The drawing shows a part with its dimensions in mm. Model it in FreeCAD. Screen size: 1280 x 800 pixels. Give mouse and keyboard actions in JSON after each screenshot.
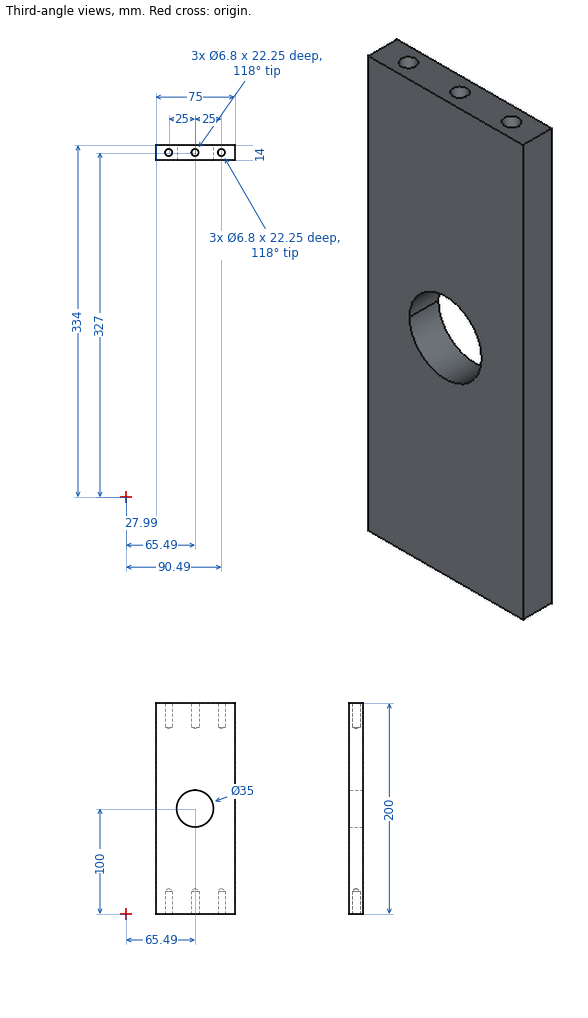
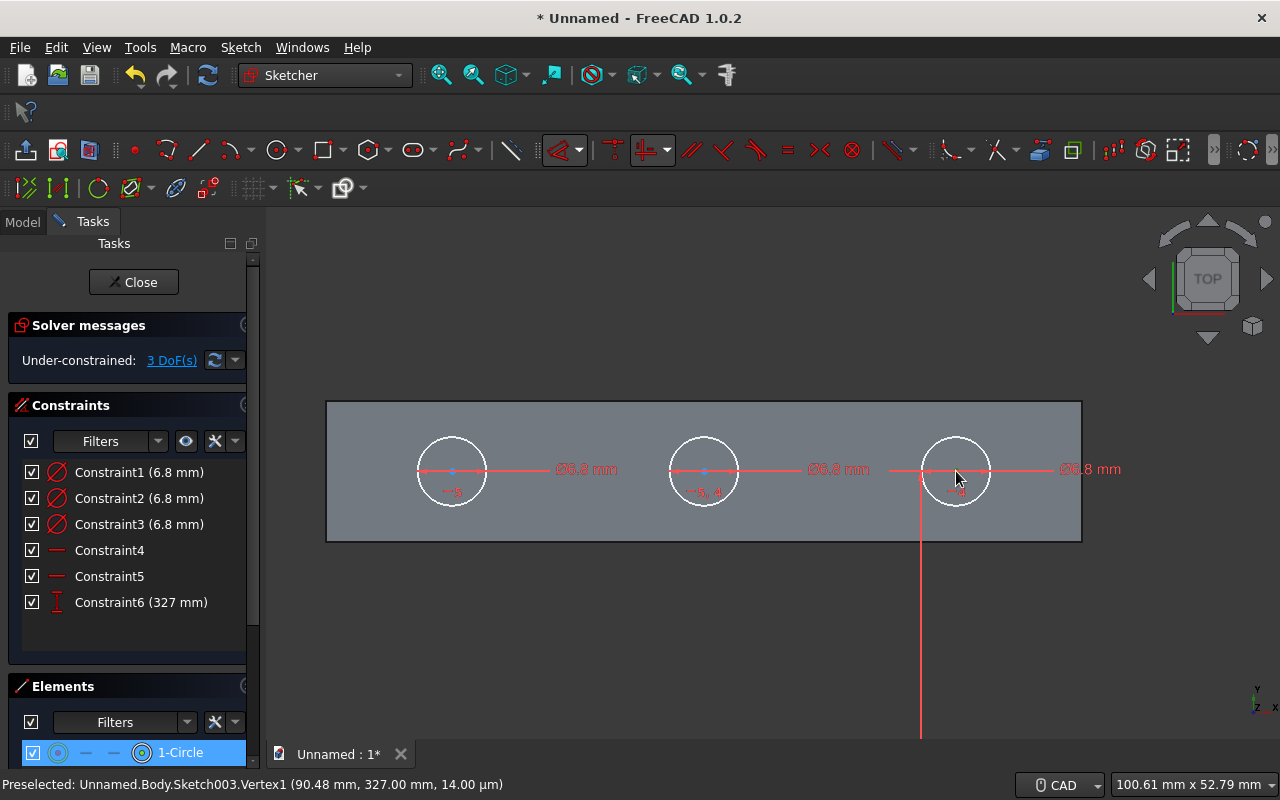
{"action": "left_click", "coordinate": [704, 471]}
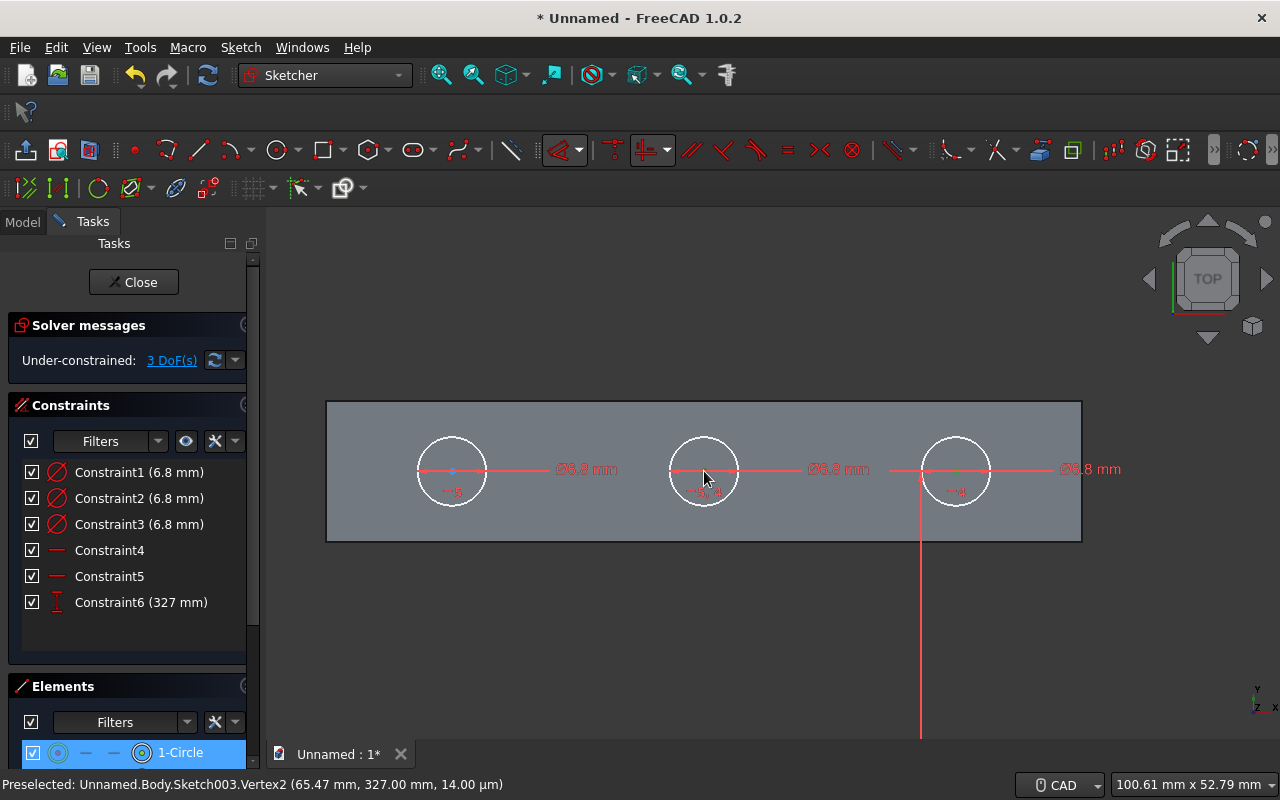
{"action": "key", "text": "l"}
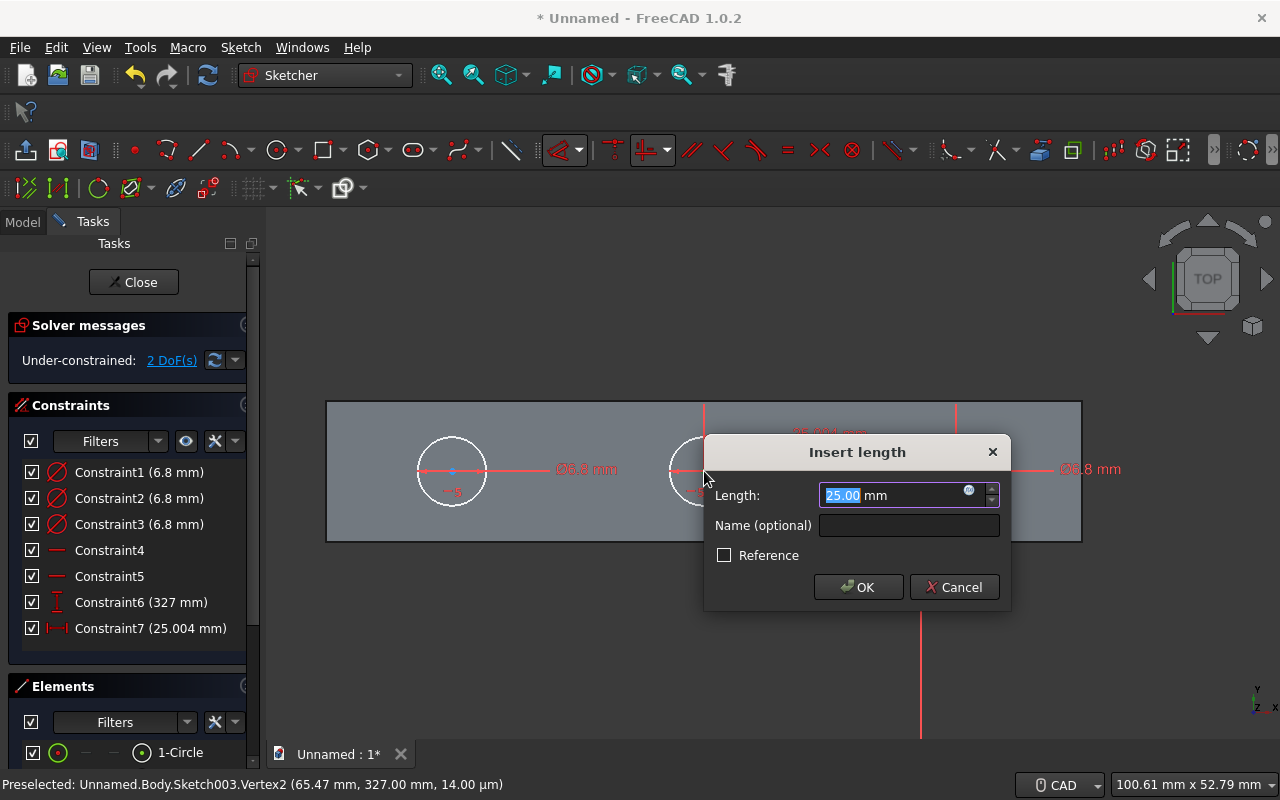
{"action": "type", "text": "25"}
{"action": "key", "text": "Return"}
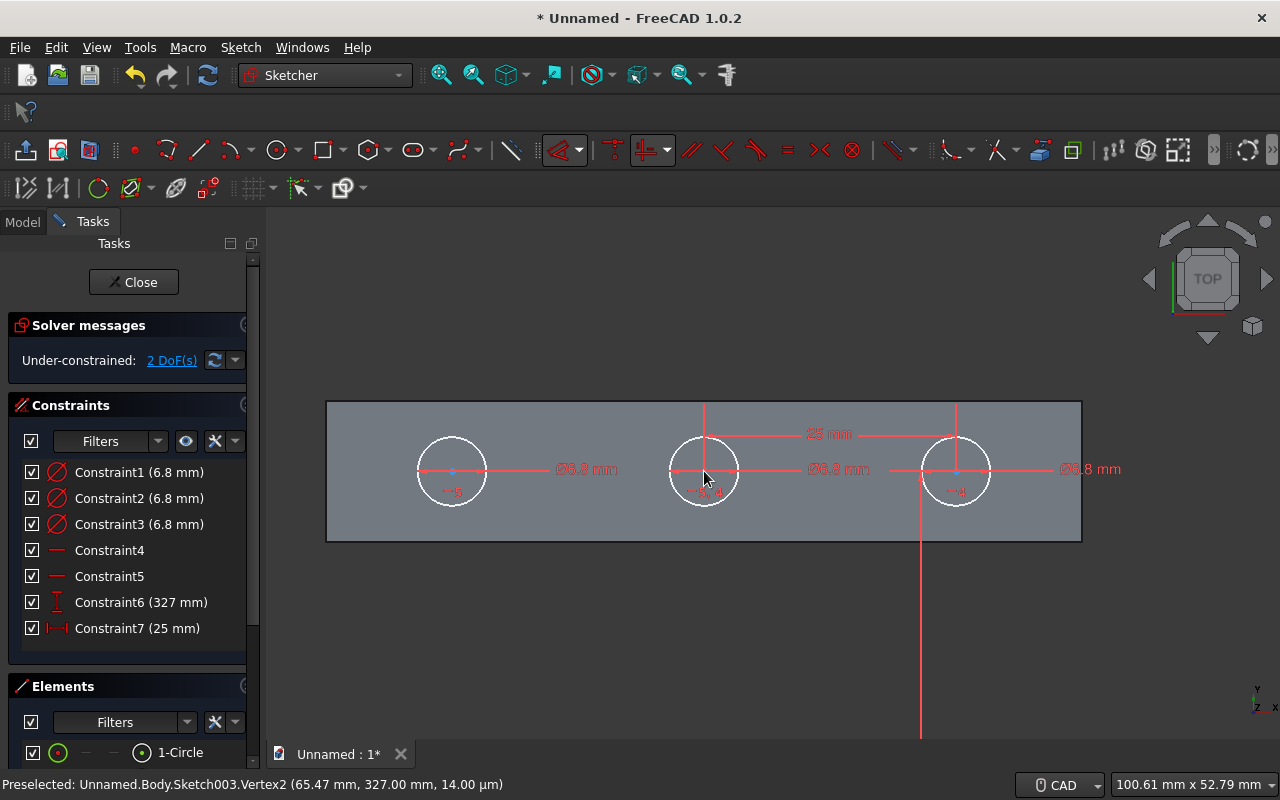
{"action": "left_click", "coordinate": [704, 471]}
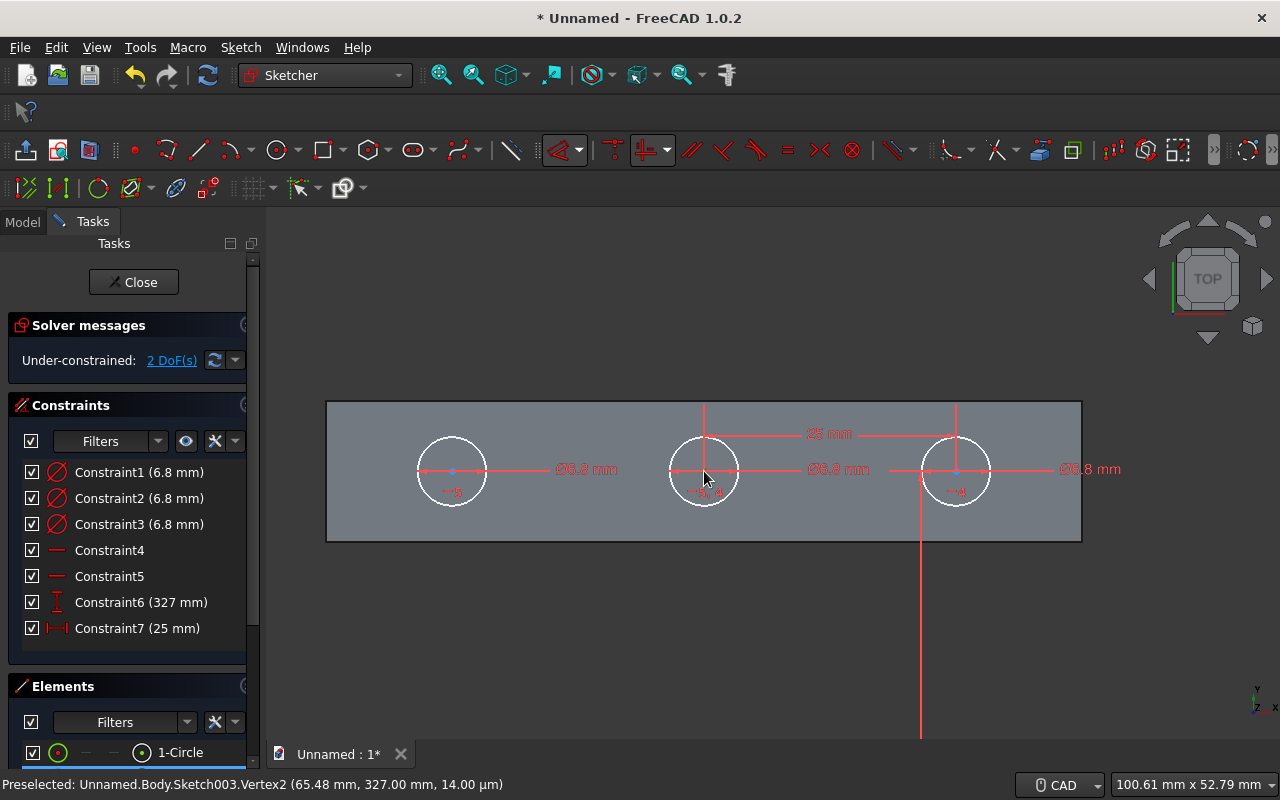
{"action": "left_click", "coordinate": [452, 471]}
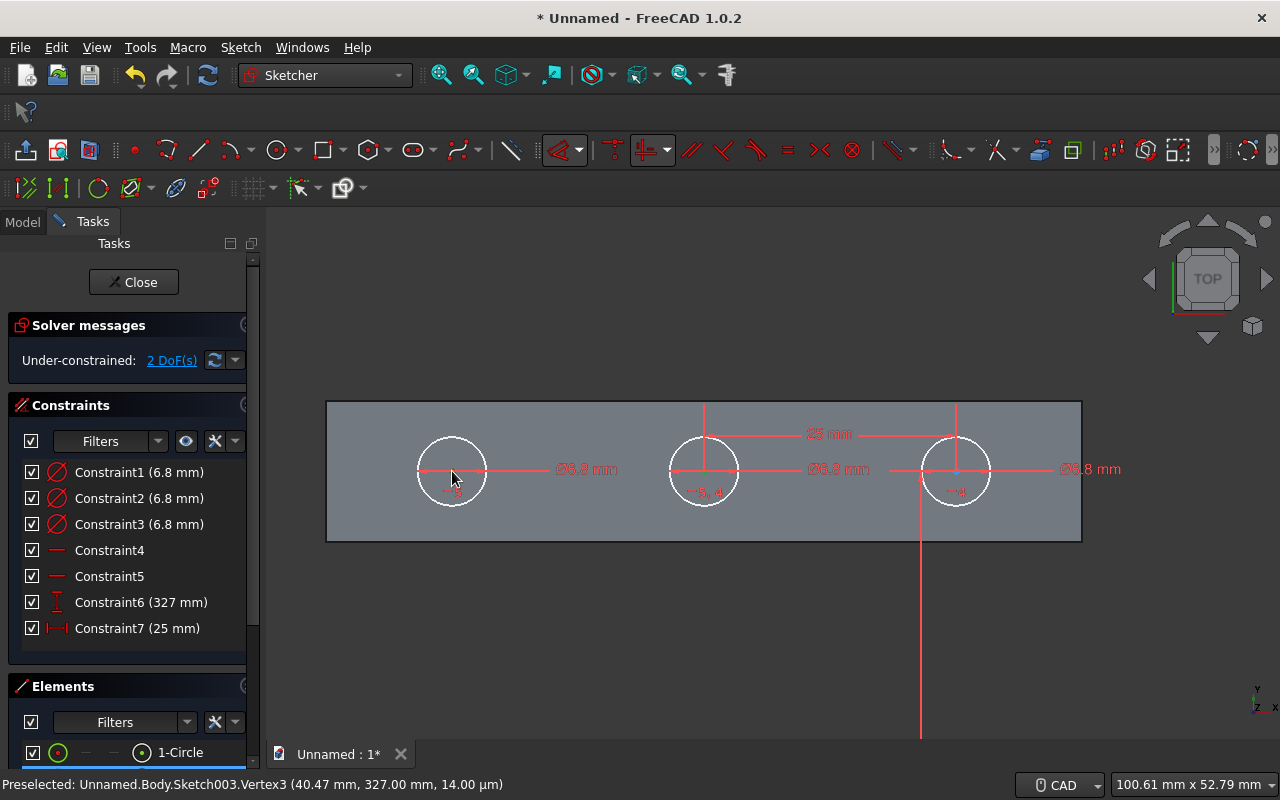
{"action": "key", "text": "l"}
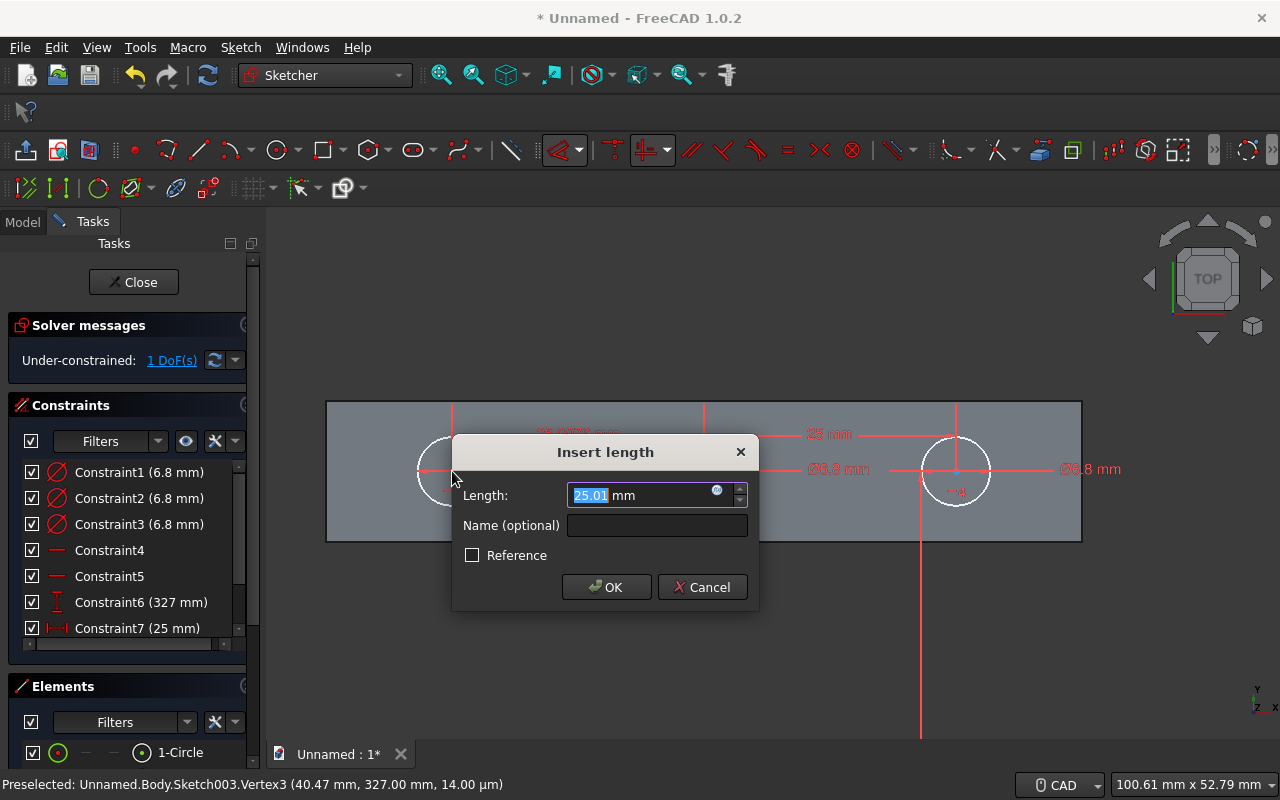
{"action": "type", "text": "25"}
{"action": "key", "text": "Return"}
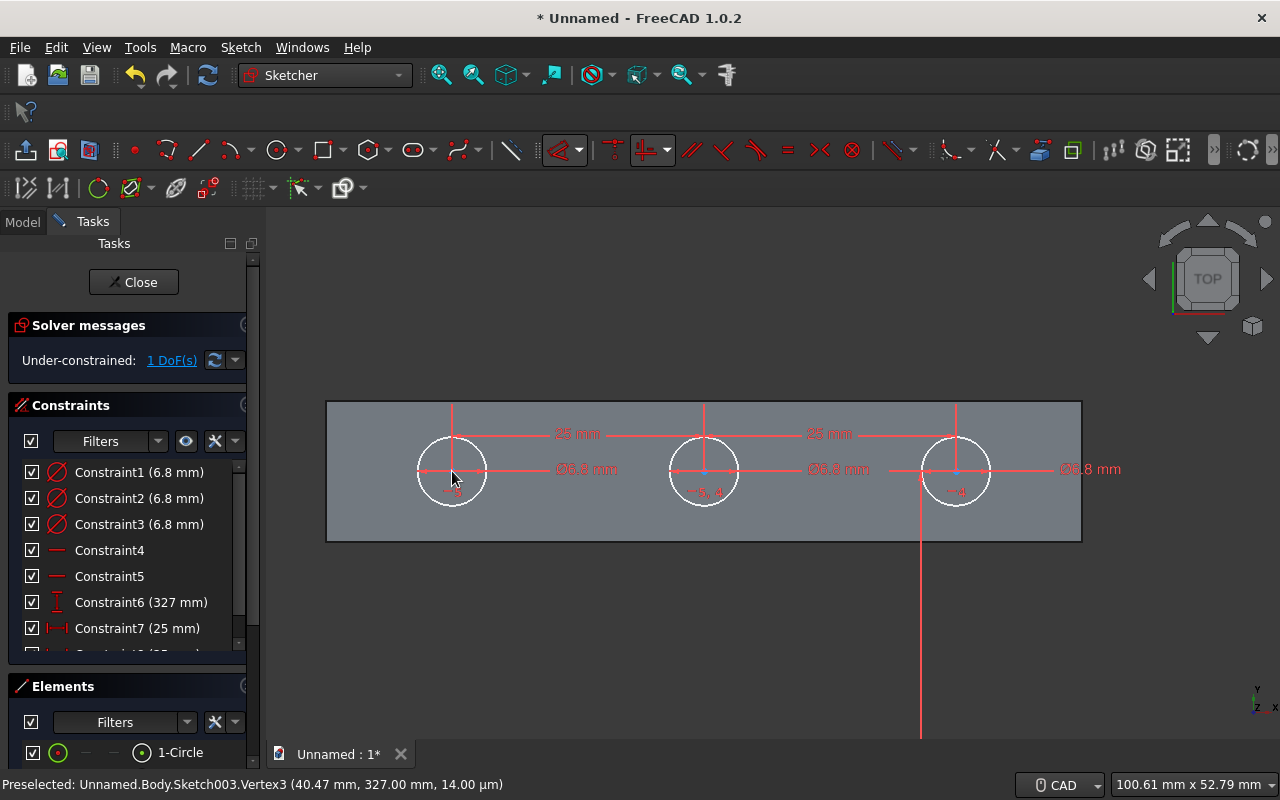
{"action": "left_click", "coordinate": [956, 471]}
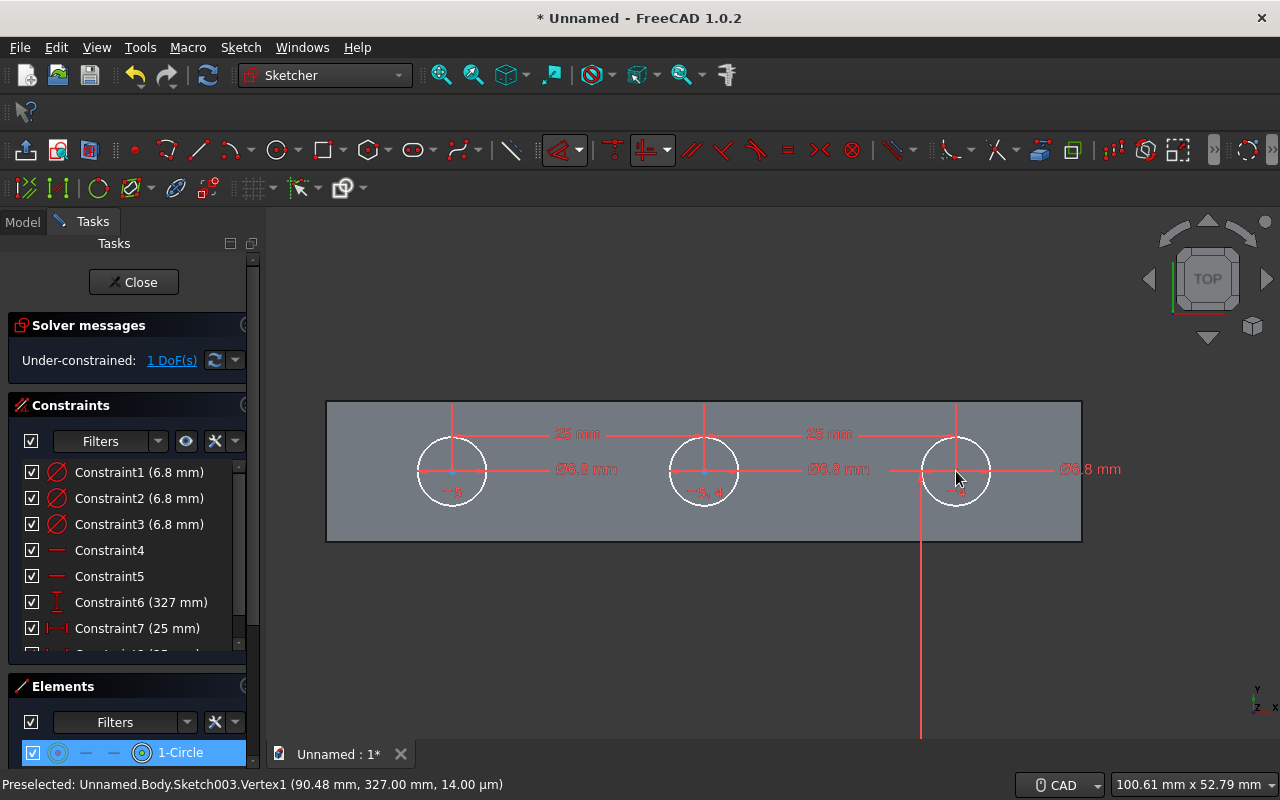
{"action": "left_click", "coordinate": [582, 150]}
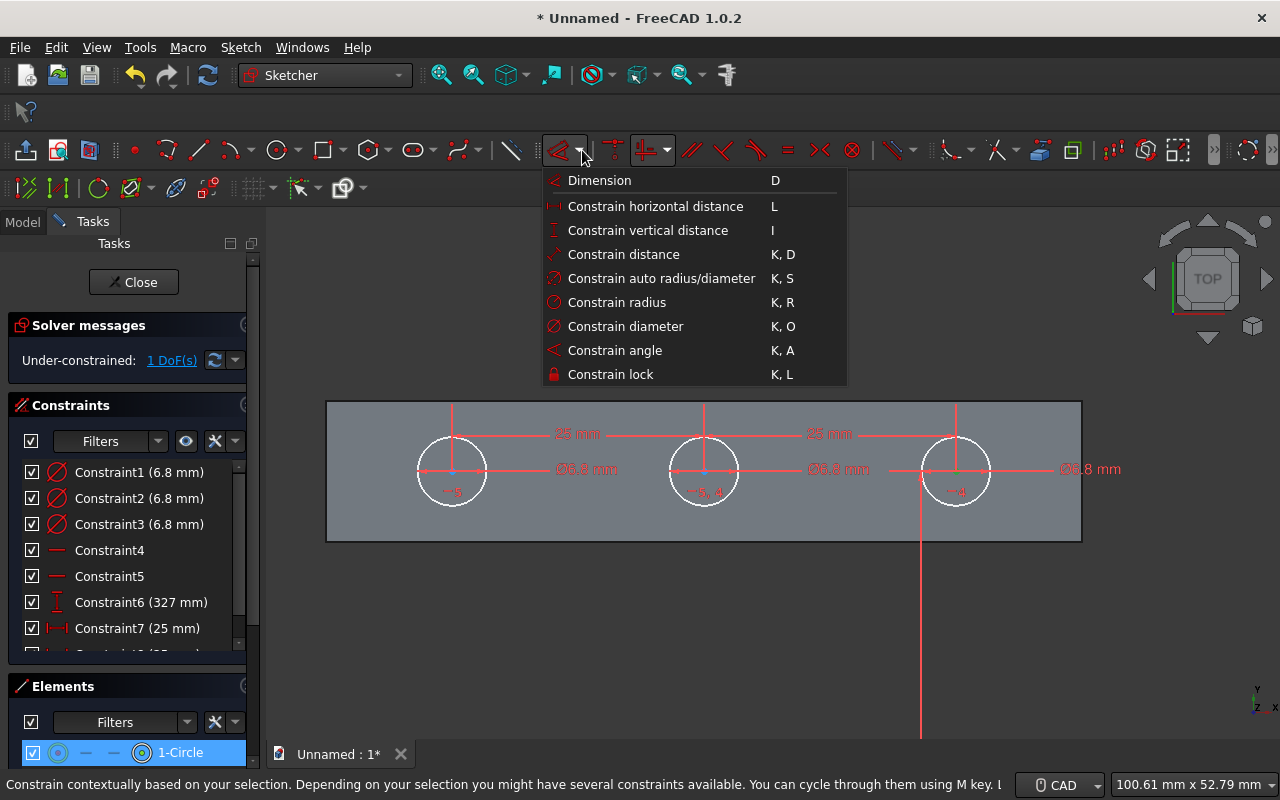
{"action": "left_click", "coordinate": [695, 206]}